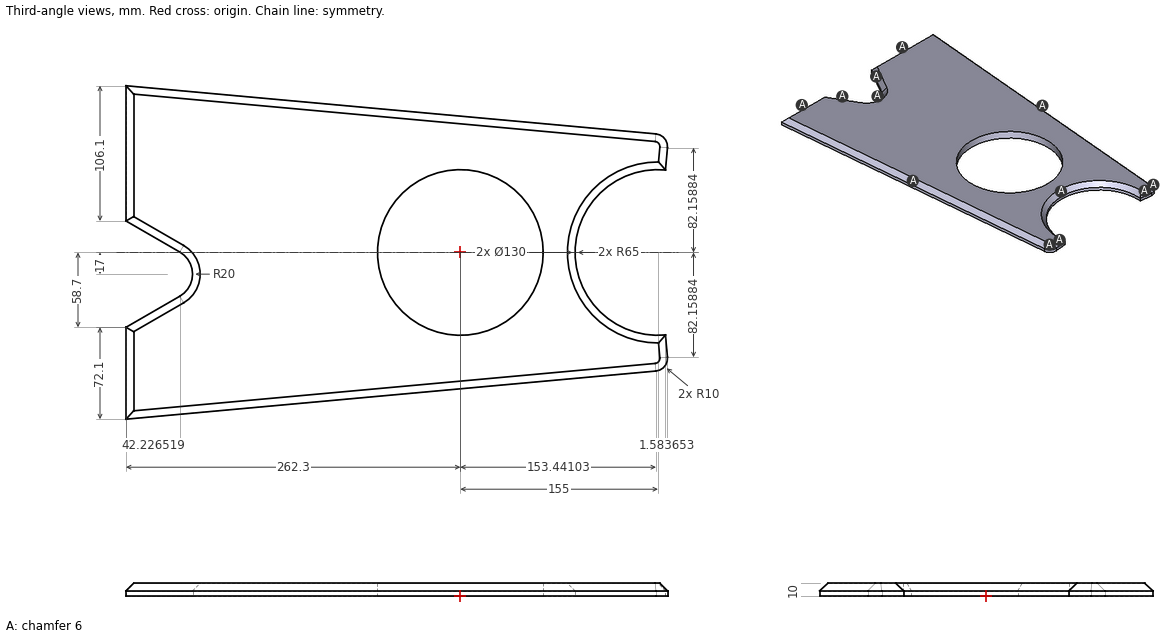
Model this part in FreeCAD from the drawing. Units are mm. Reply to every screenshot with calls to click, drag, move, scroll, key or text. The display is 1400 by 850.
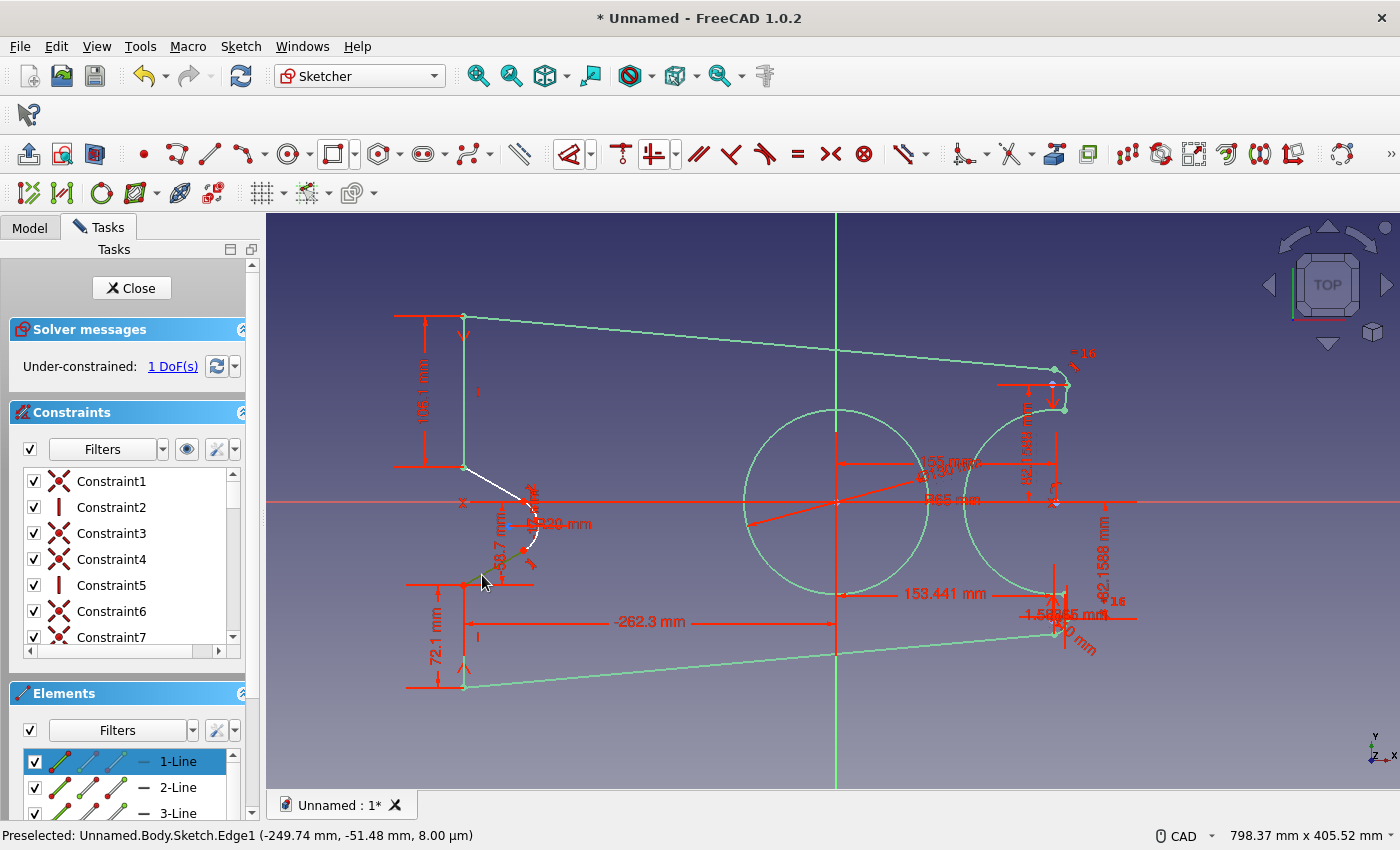
key(l)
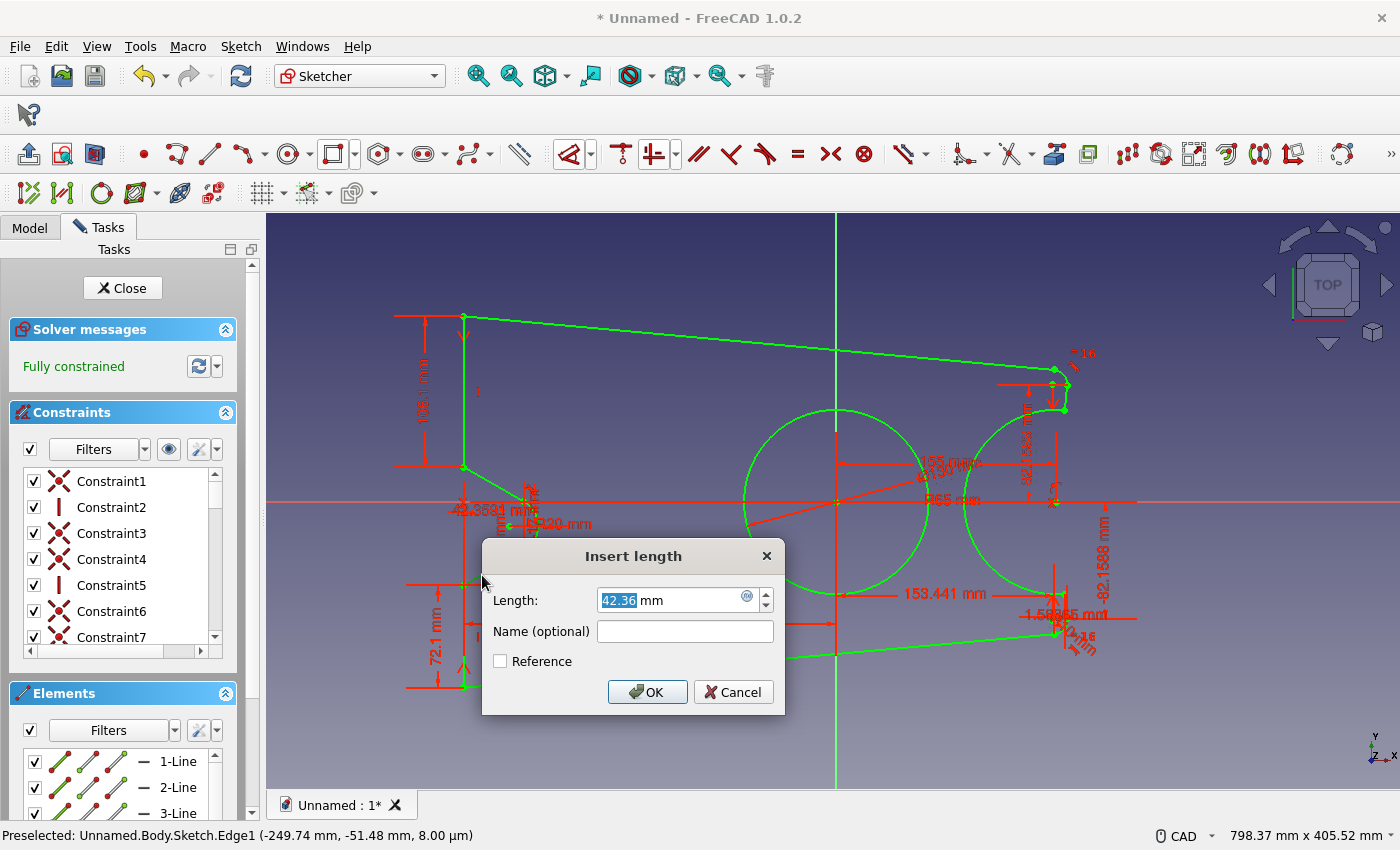
text(42.226519)
key(Return)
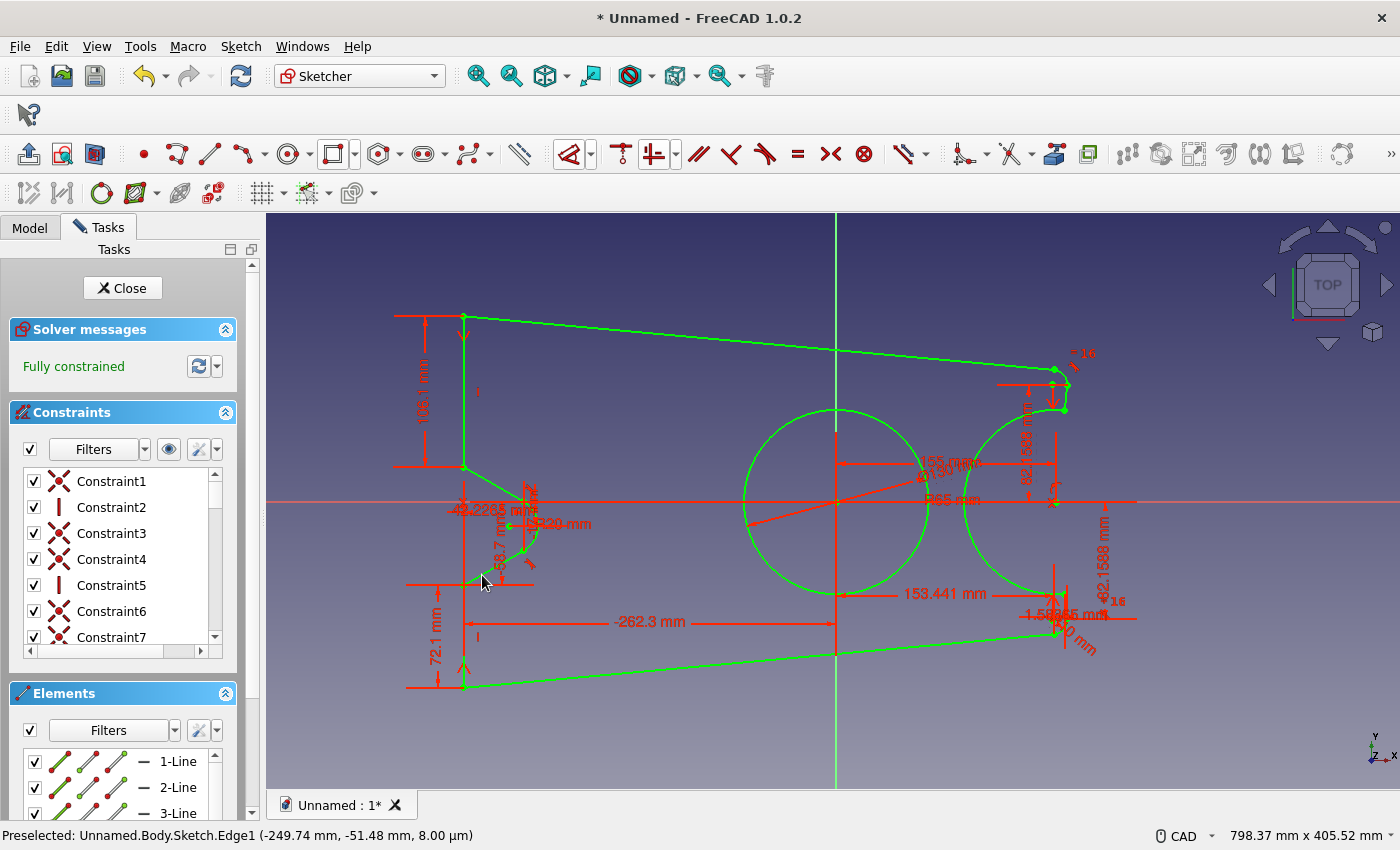
click(123, 288)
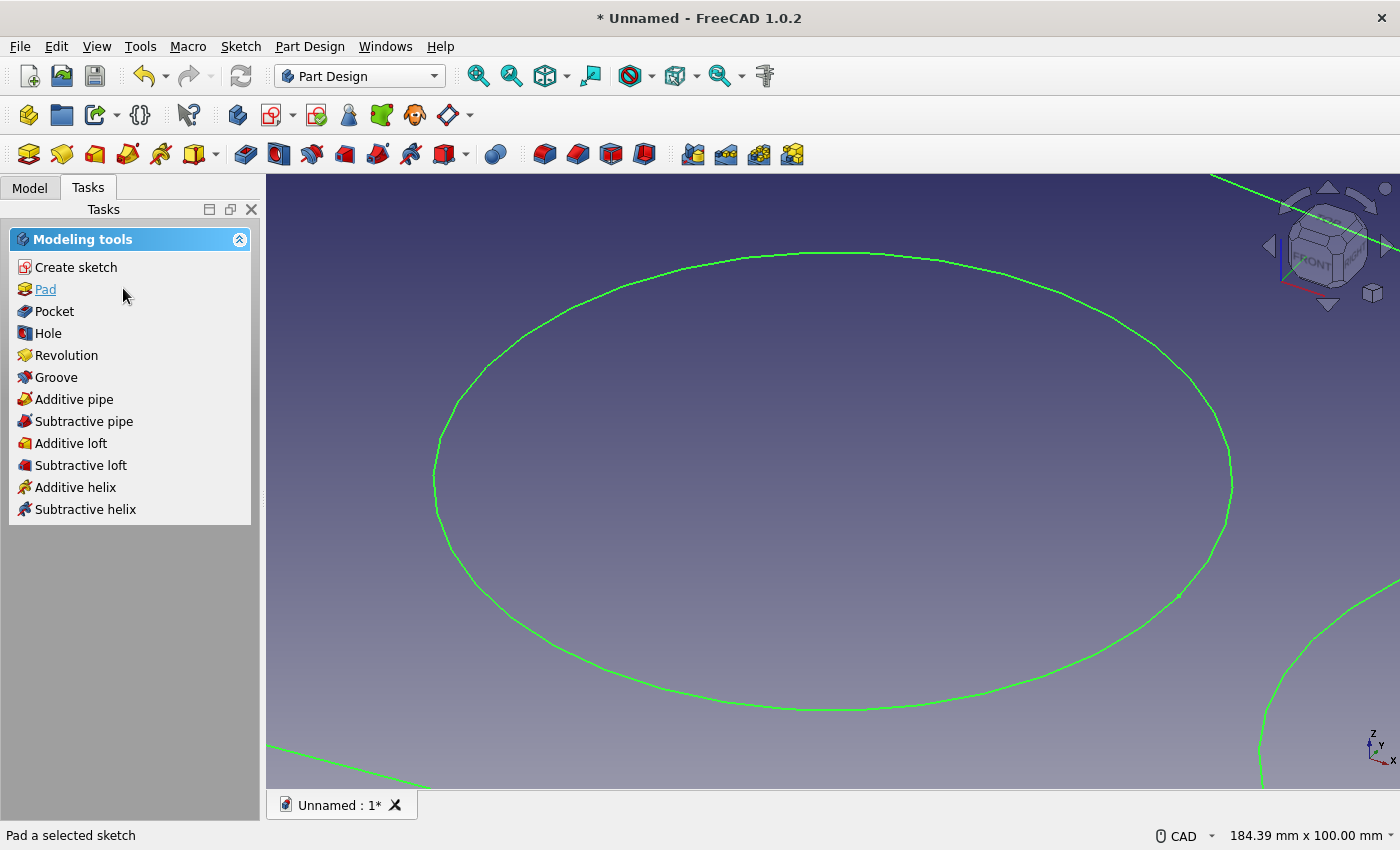
click(29, 154)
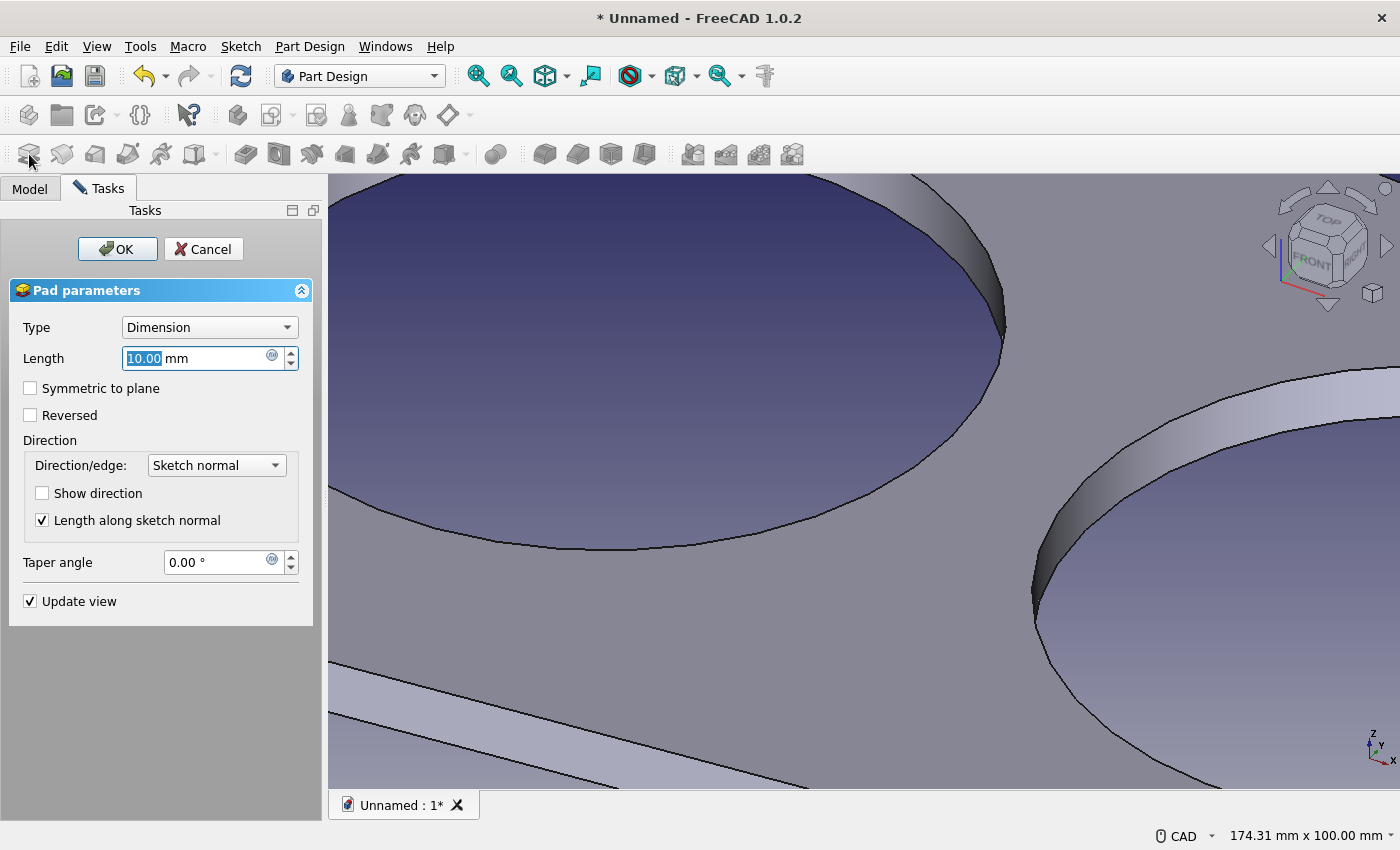
text(10)
key(Tab)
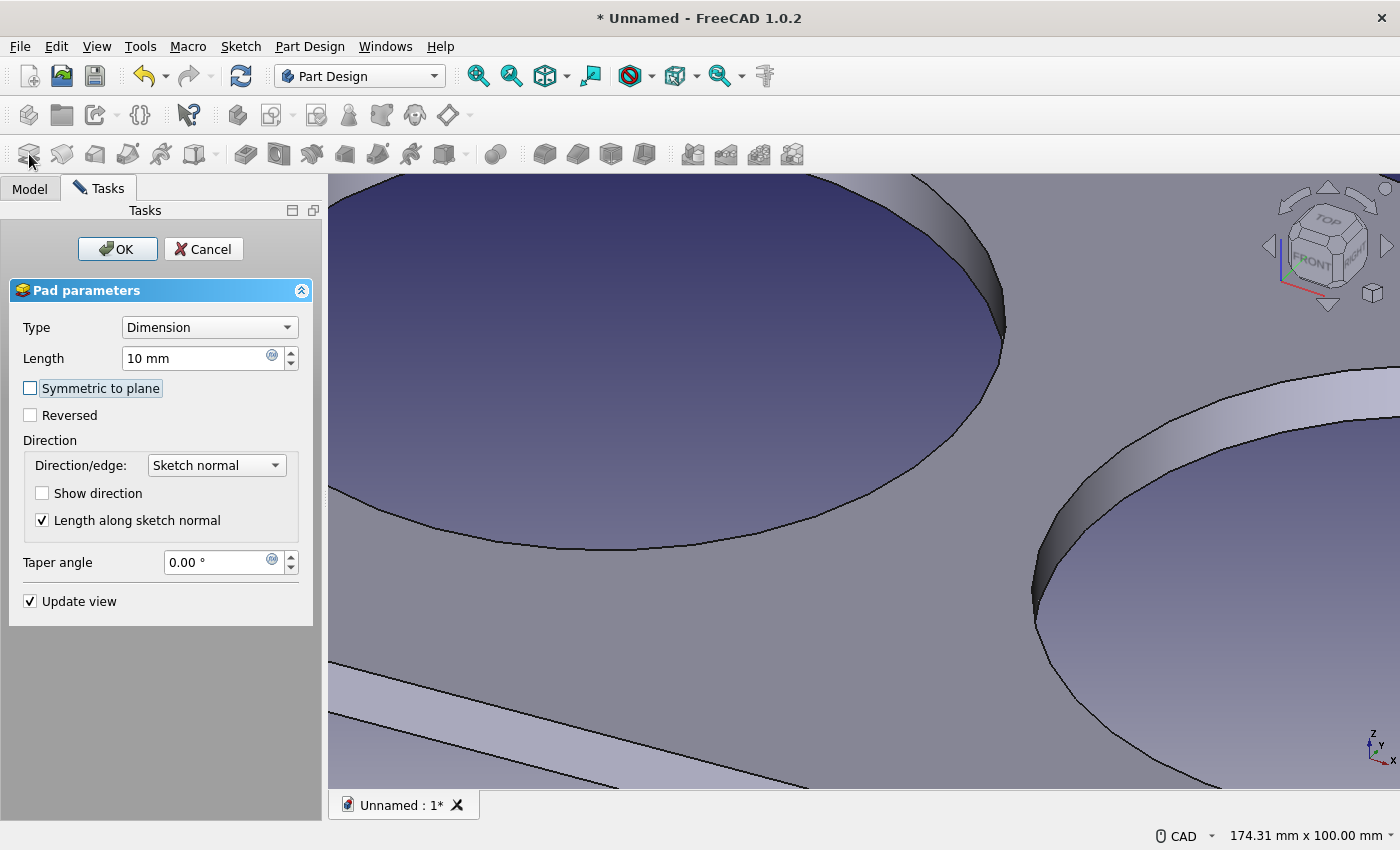
click(118, 249)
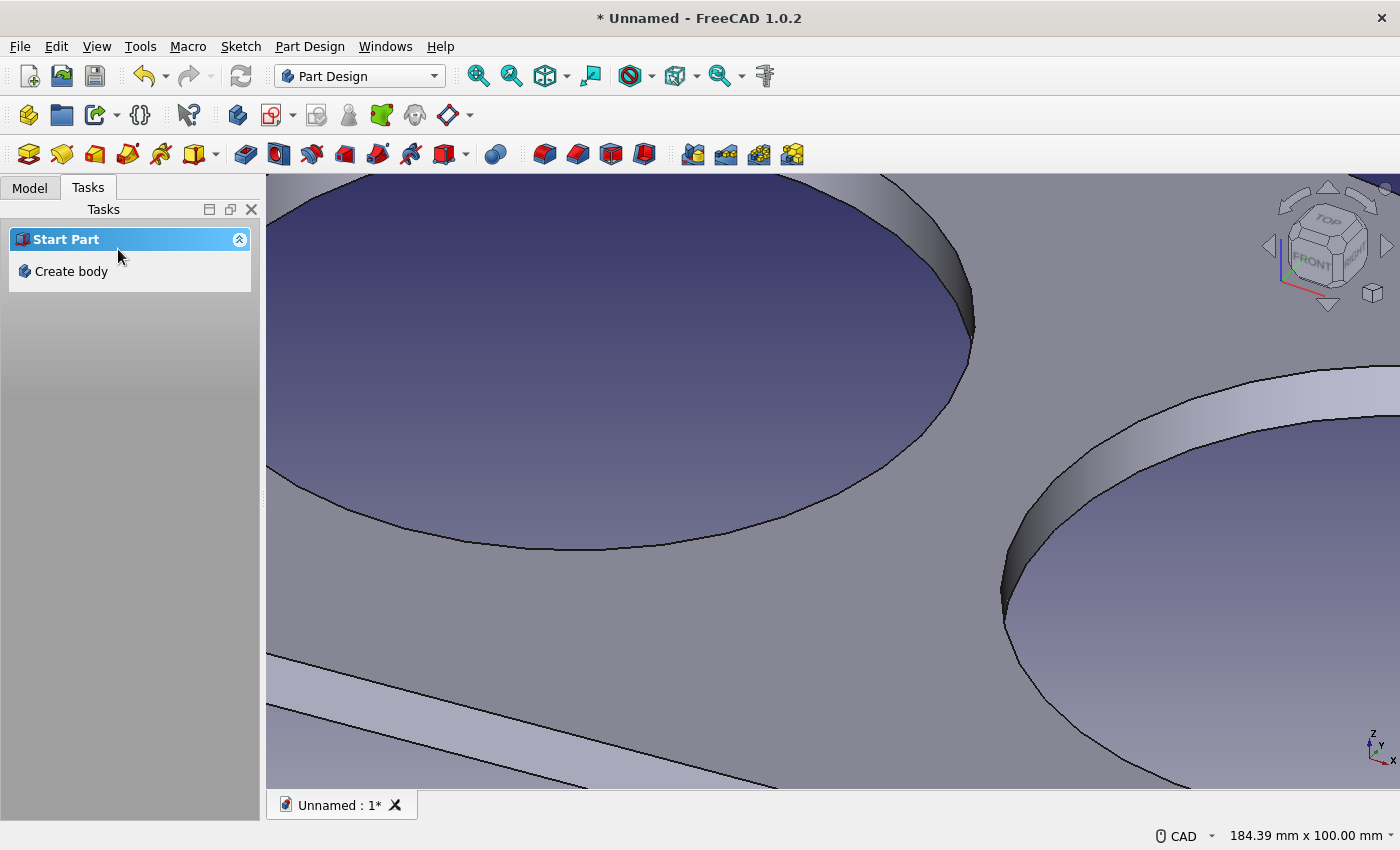
click(479, 76)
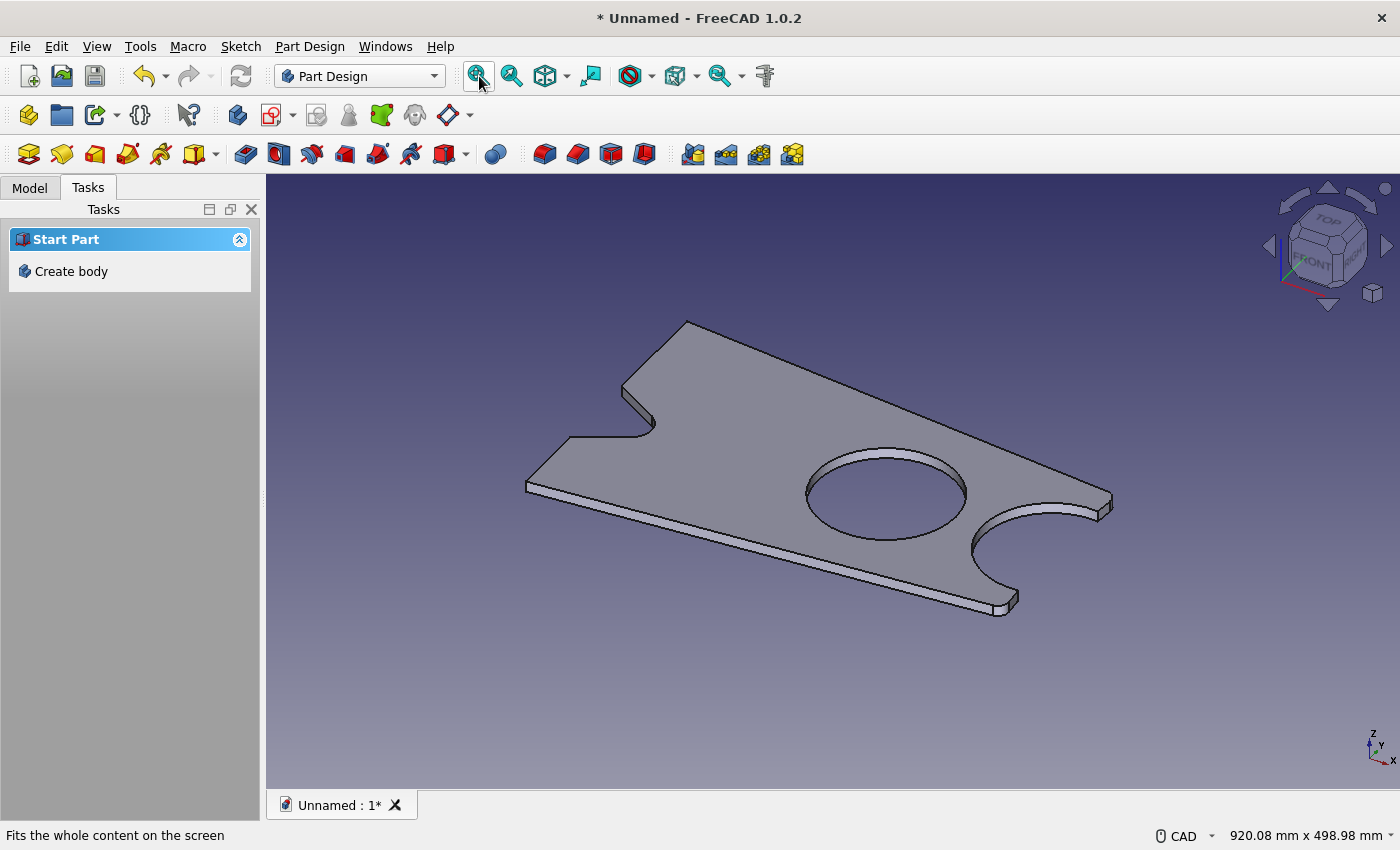
click(1002, 604)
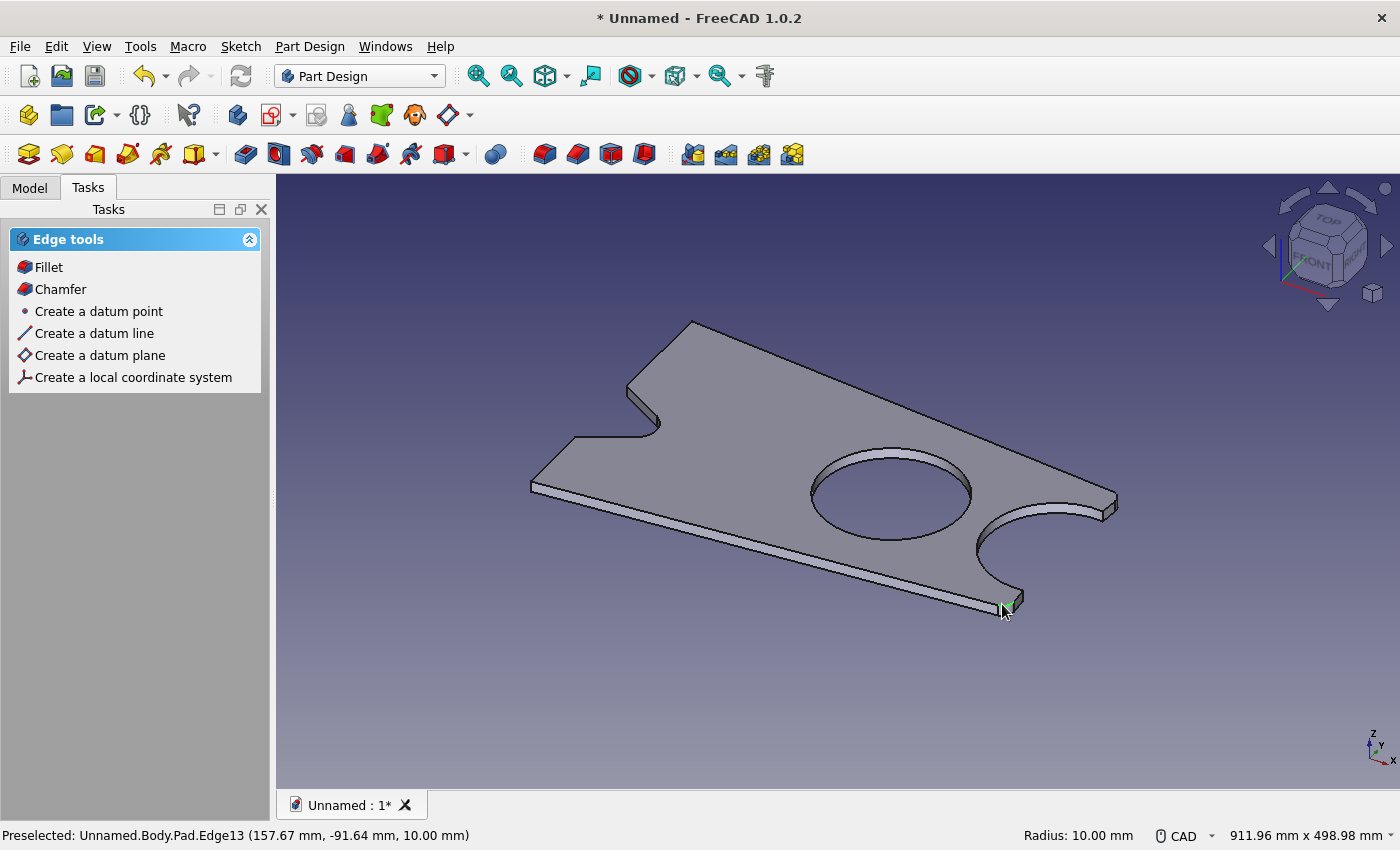
click(1019, 595, ctrl)